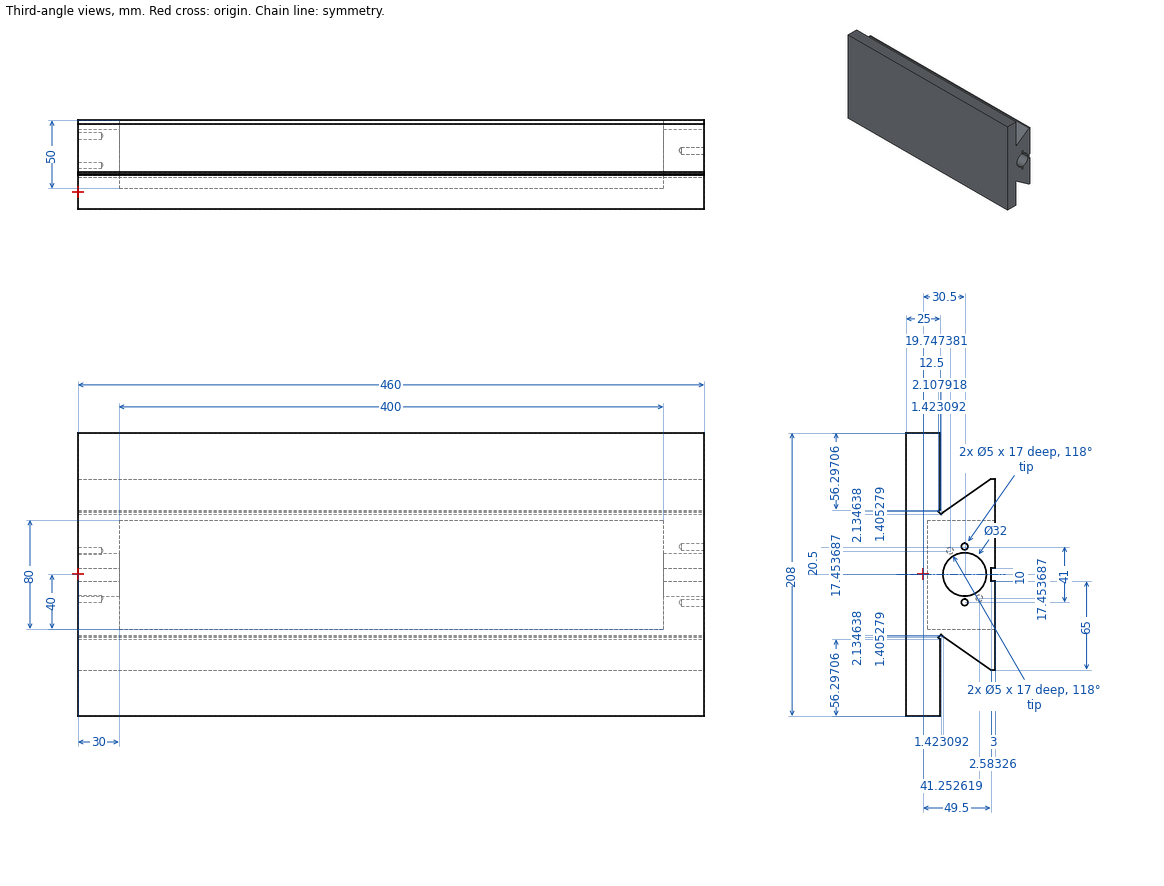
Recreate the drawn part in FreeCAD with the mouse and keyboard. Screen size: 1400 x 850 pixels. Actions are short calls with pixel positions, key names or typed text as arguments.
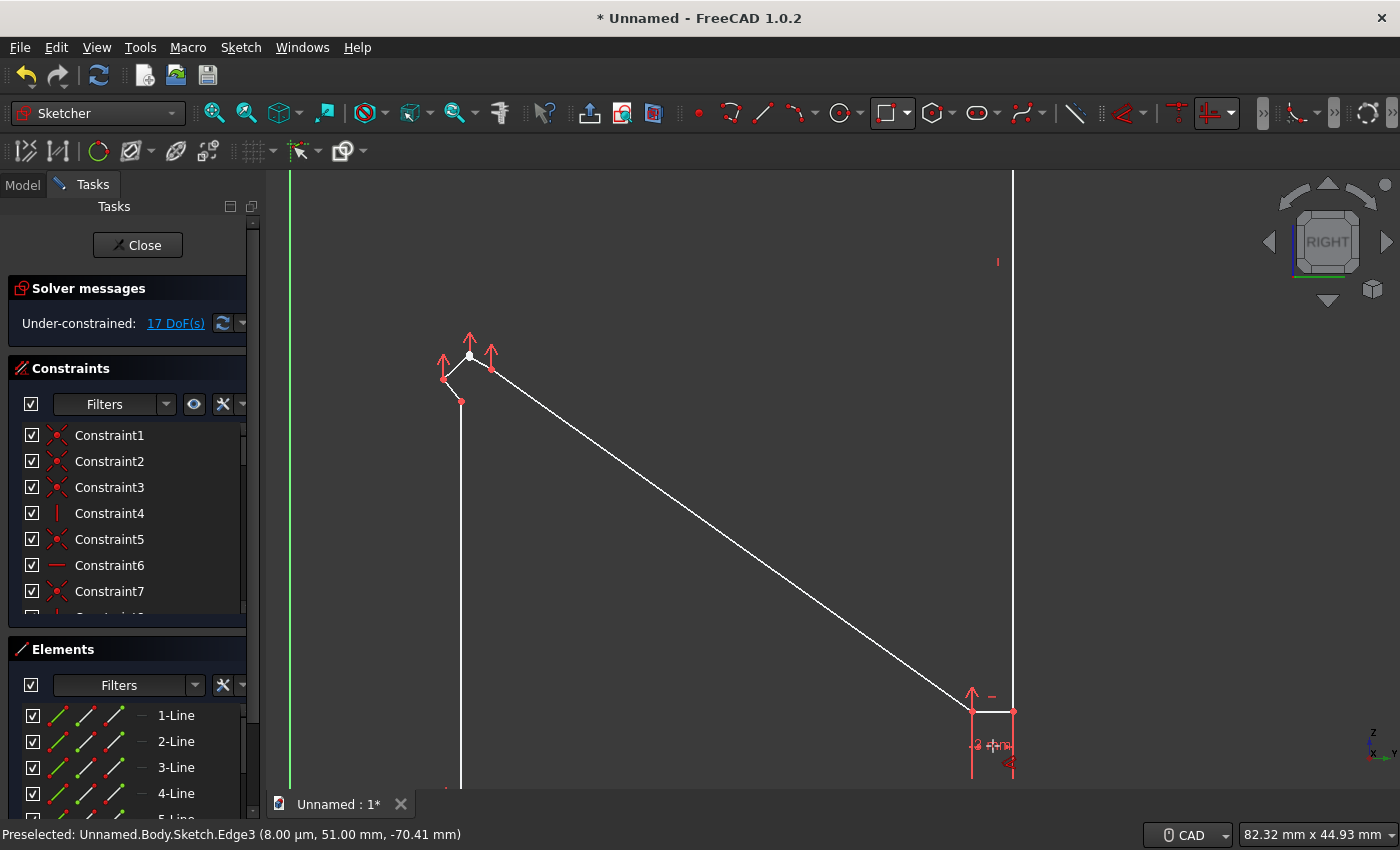
scroll(796, 595, down, 10)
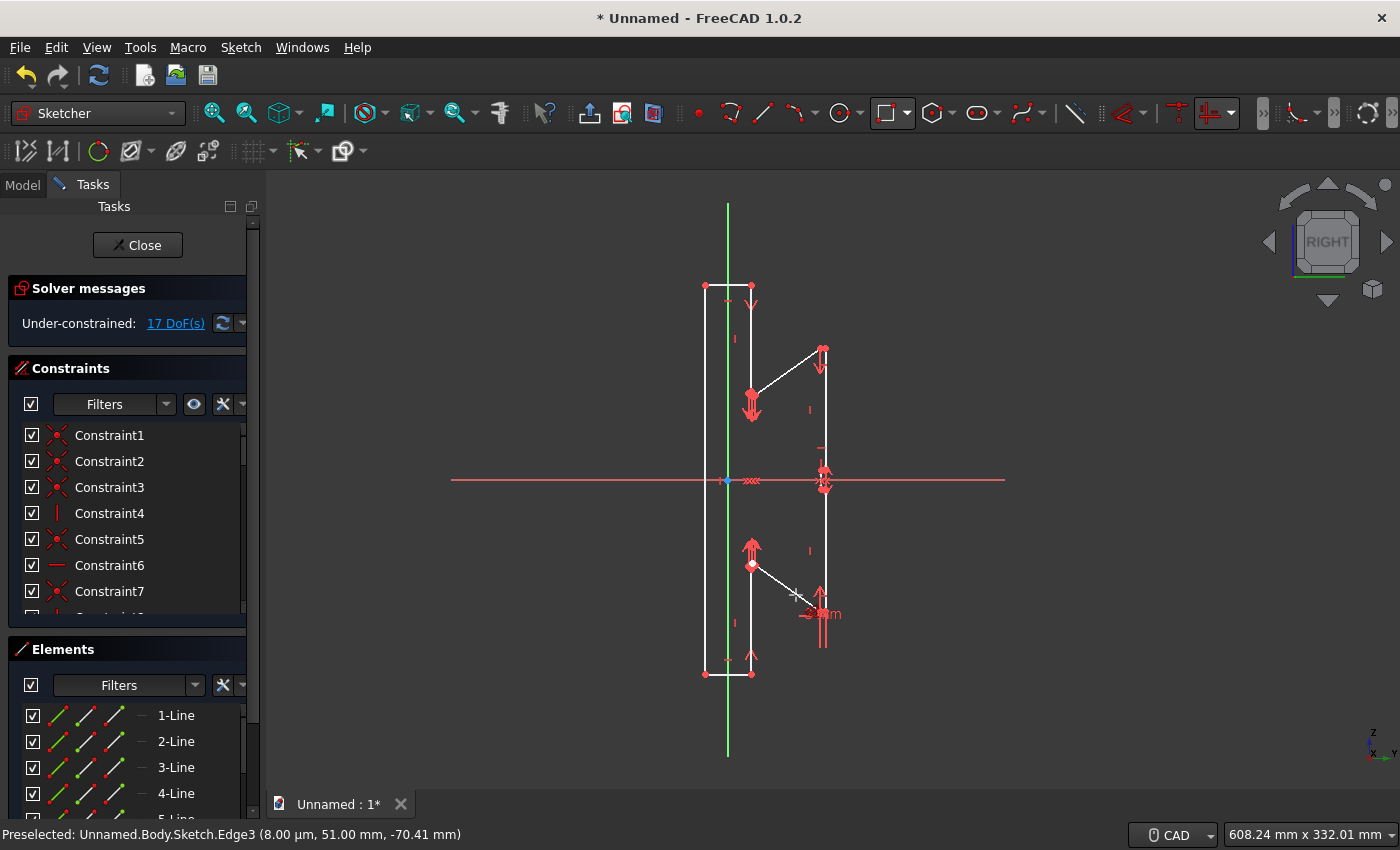
click(826, 575)
click(860, 551)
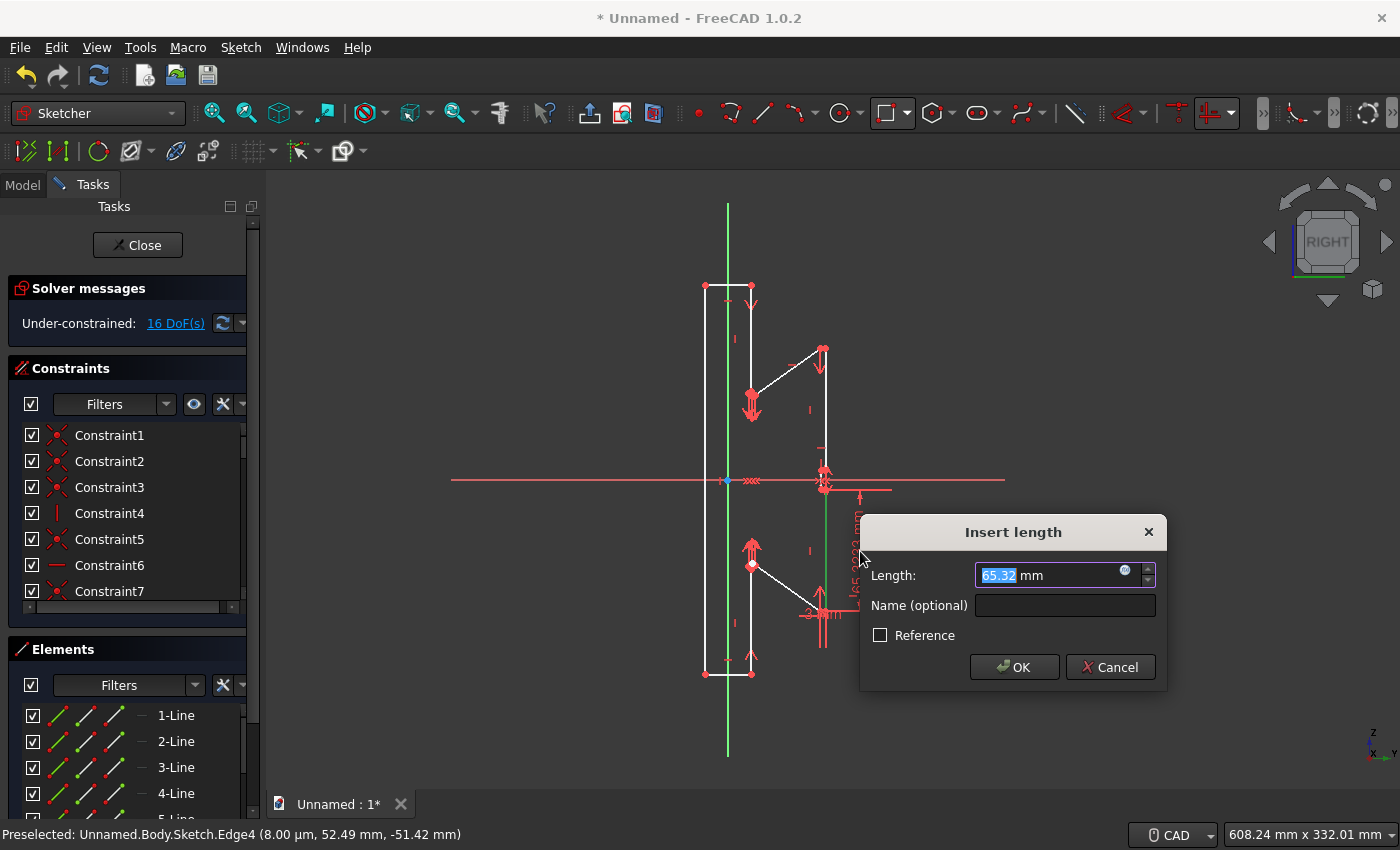
text(65)
key(Return)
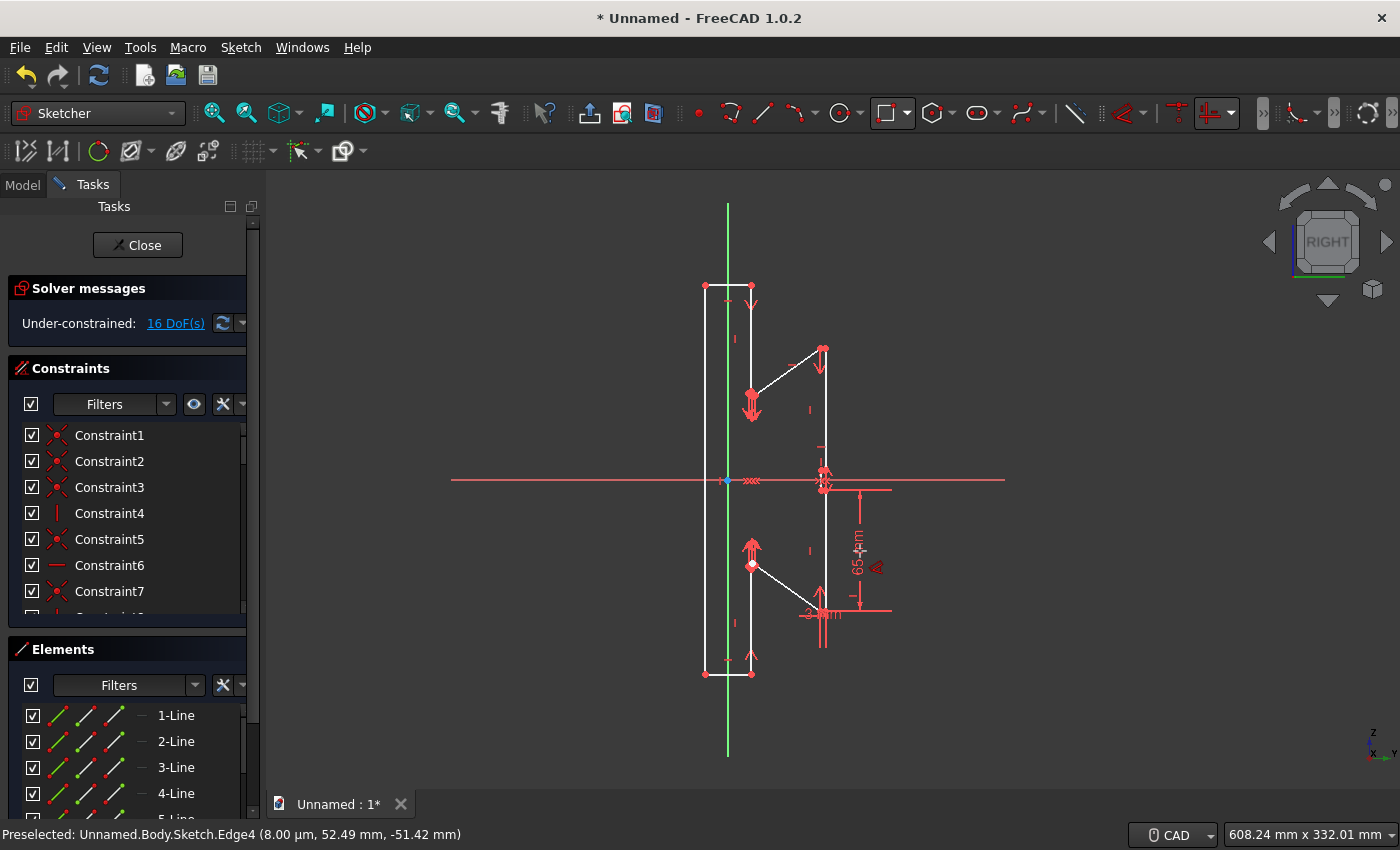
scroll(821, 480, up, 4)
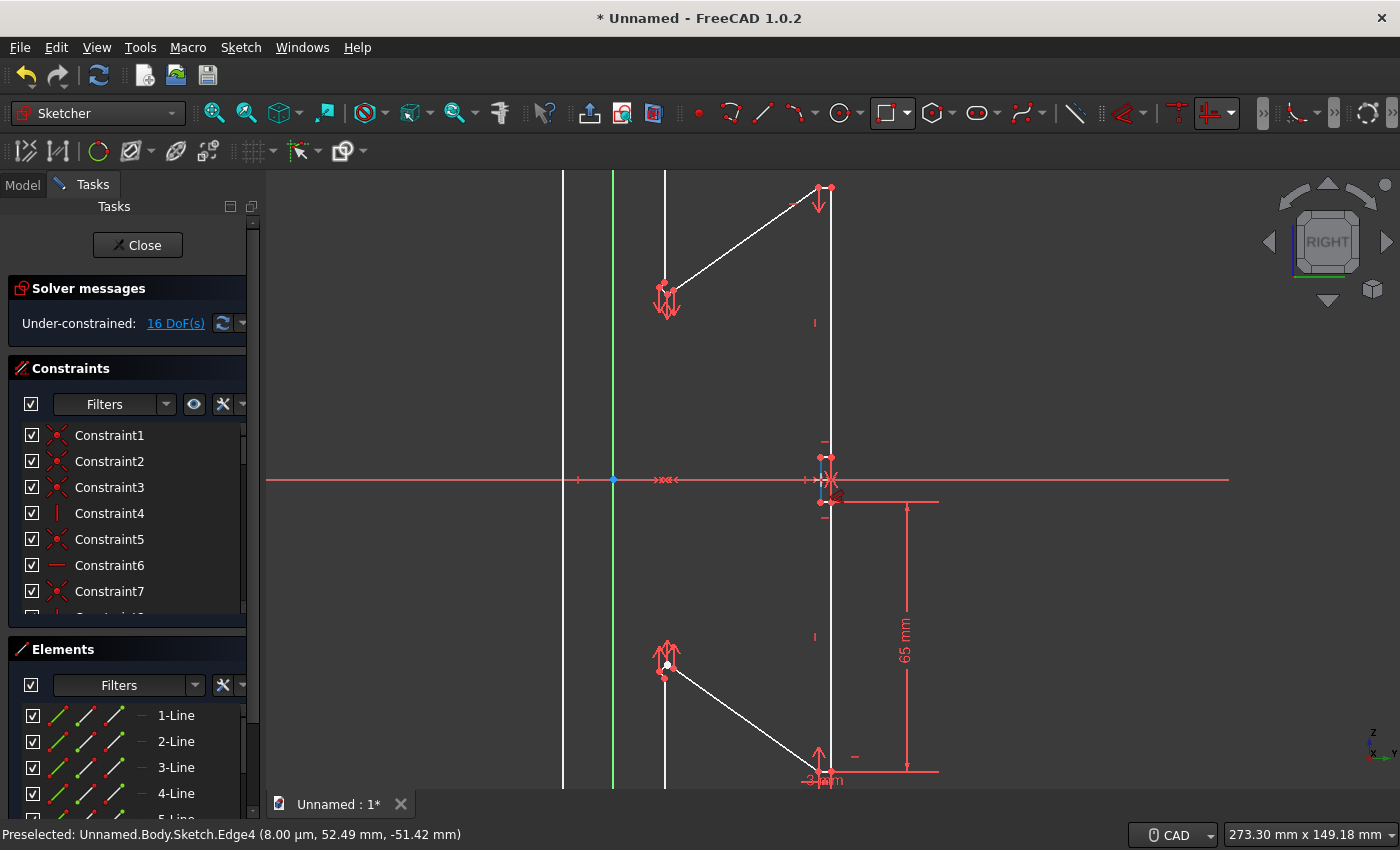
click(821, 480)
click(855, 464)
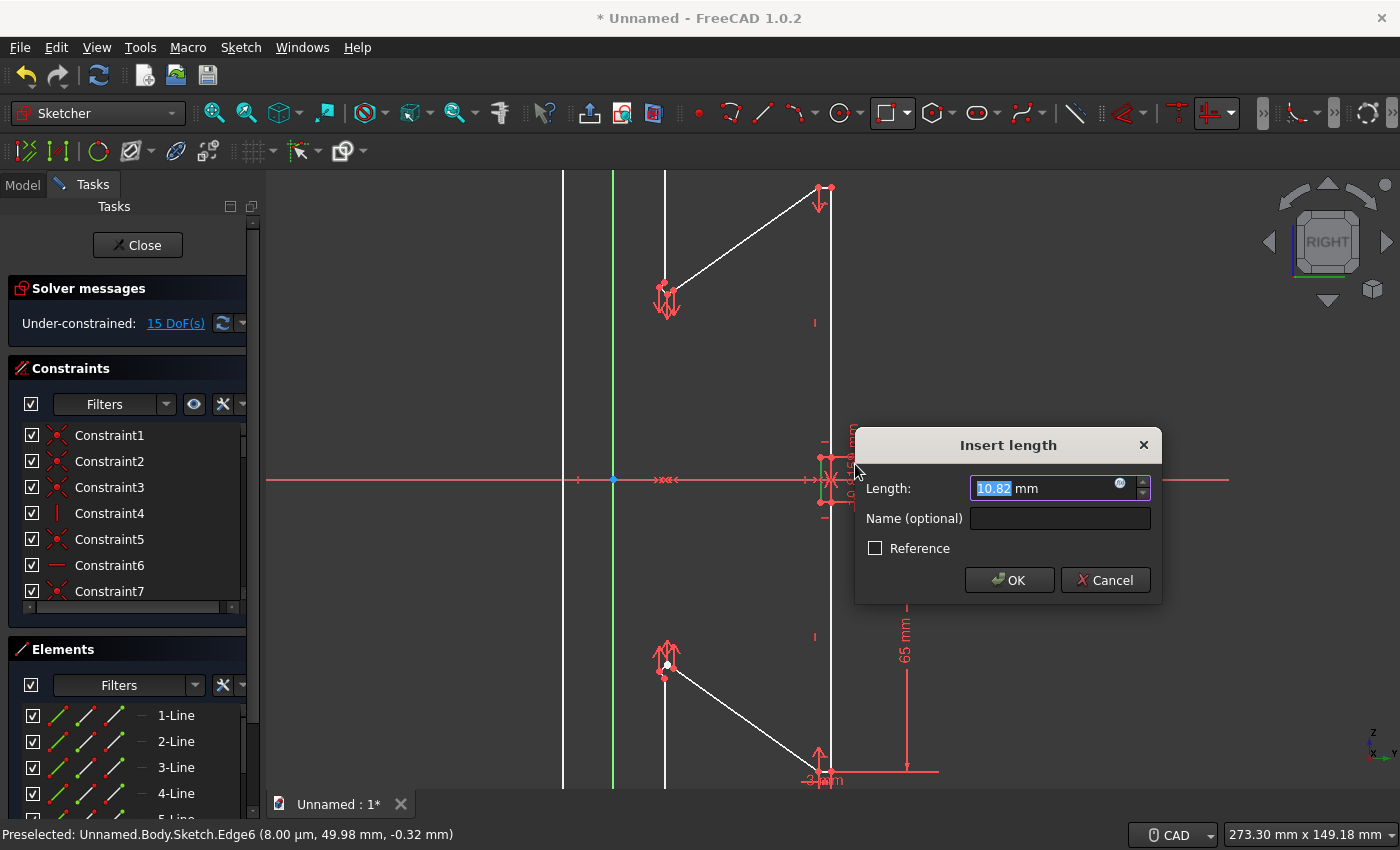
text(10)
key(Return)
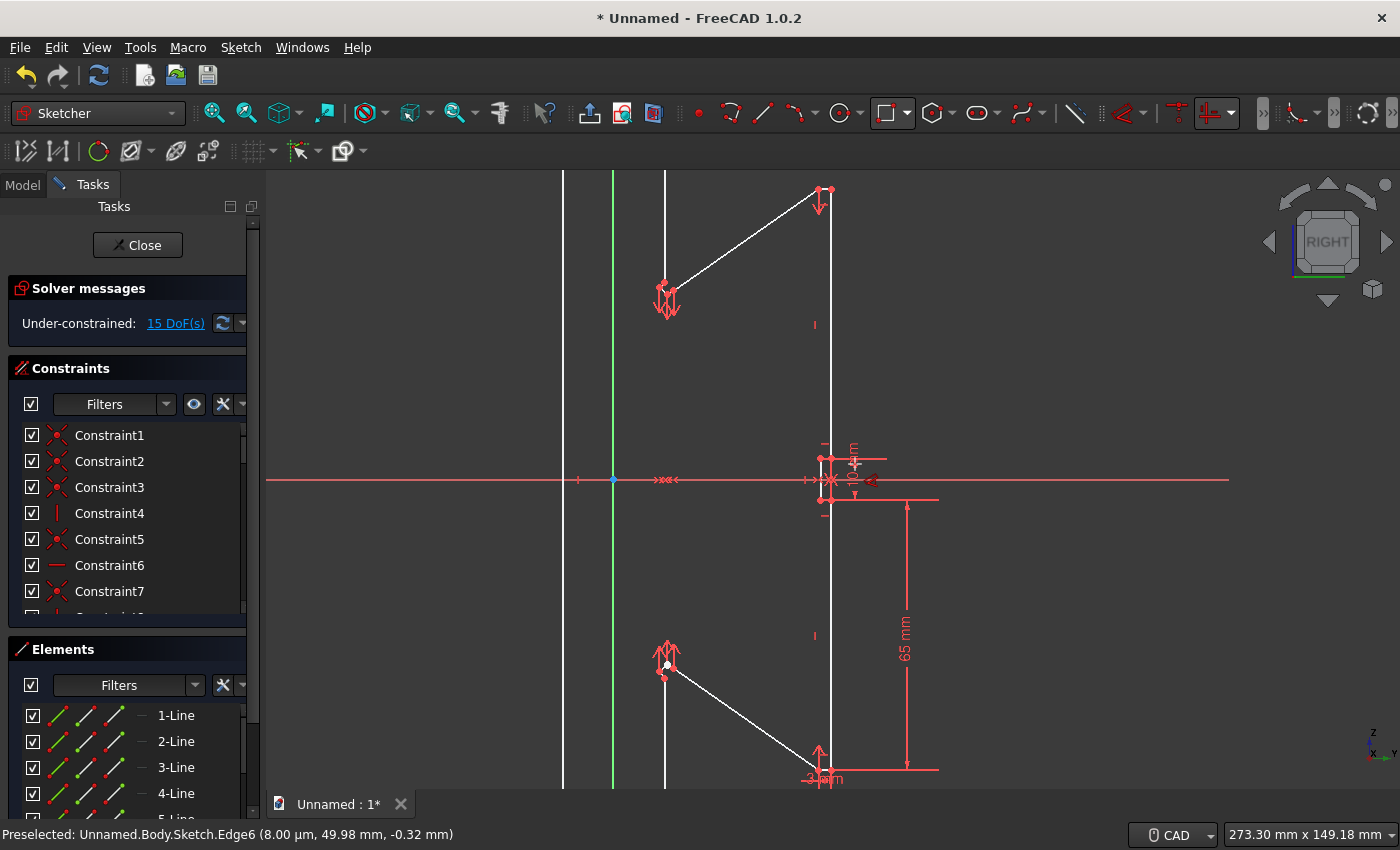
scroll(820, 479, down, 4)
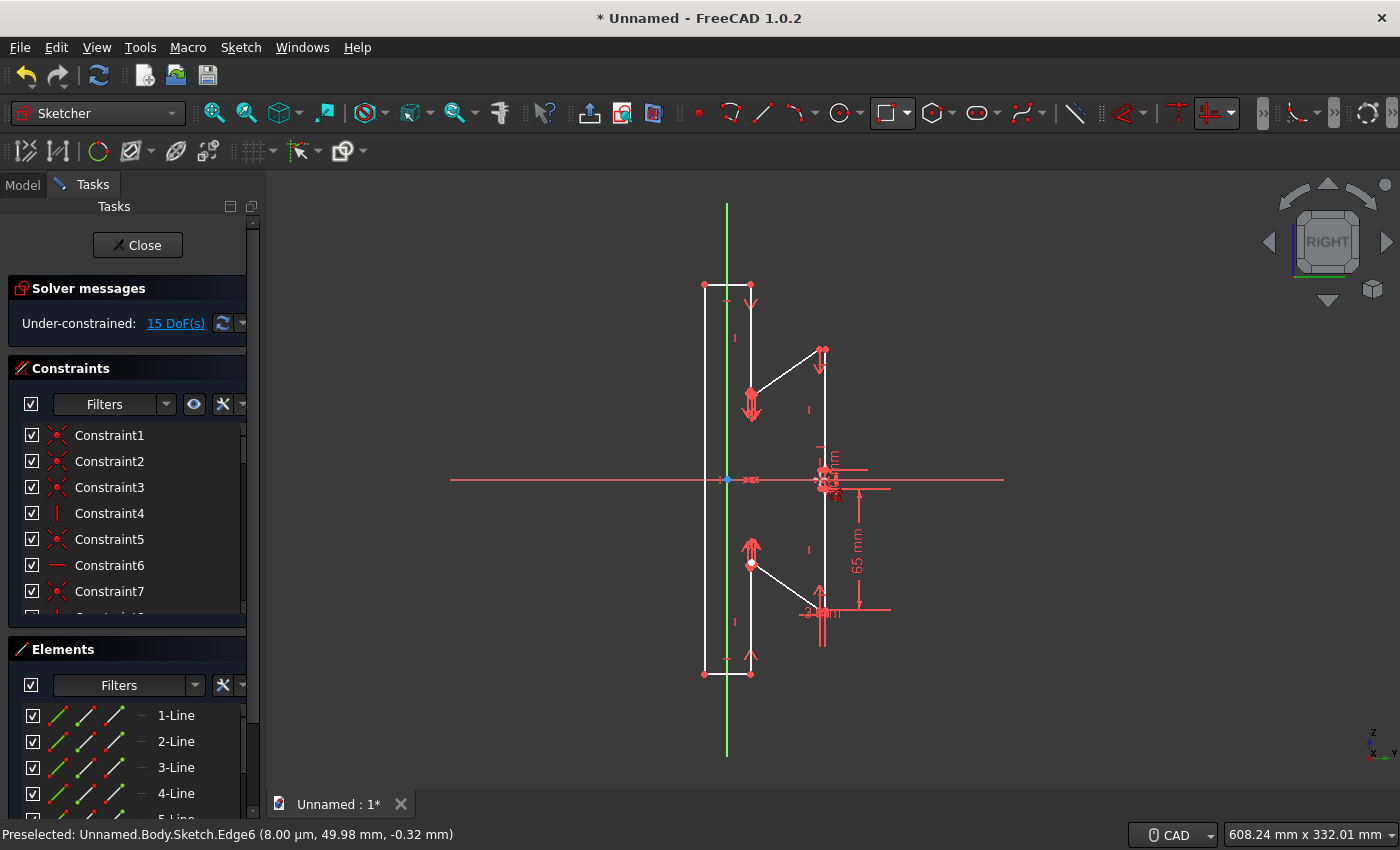
scroll(737, 285, up, 2)